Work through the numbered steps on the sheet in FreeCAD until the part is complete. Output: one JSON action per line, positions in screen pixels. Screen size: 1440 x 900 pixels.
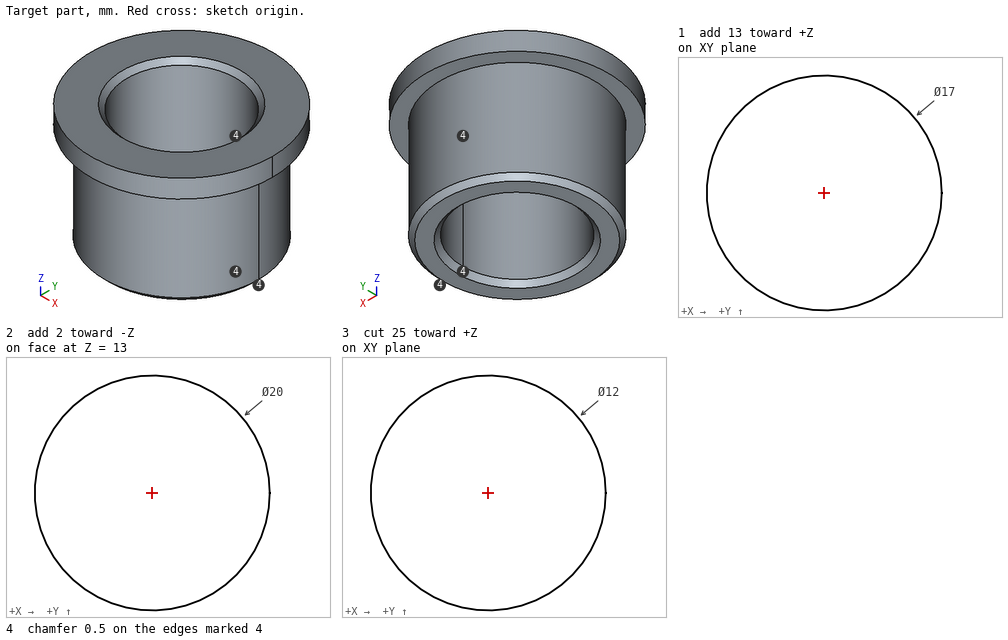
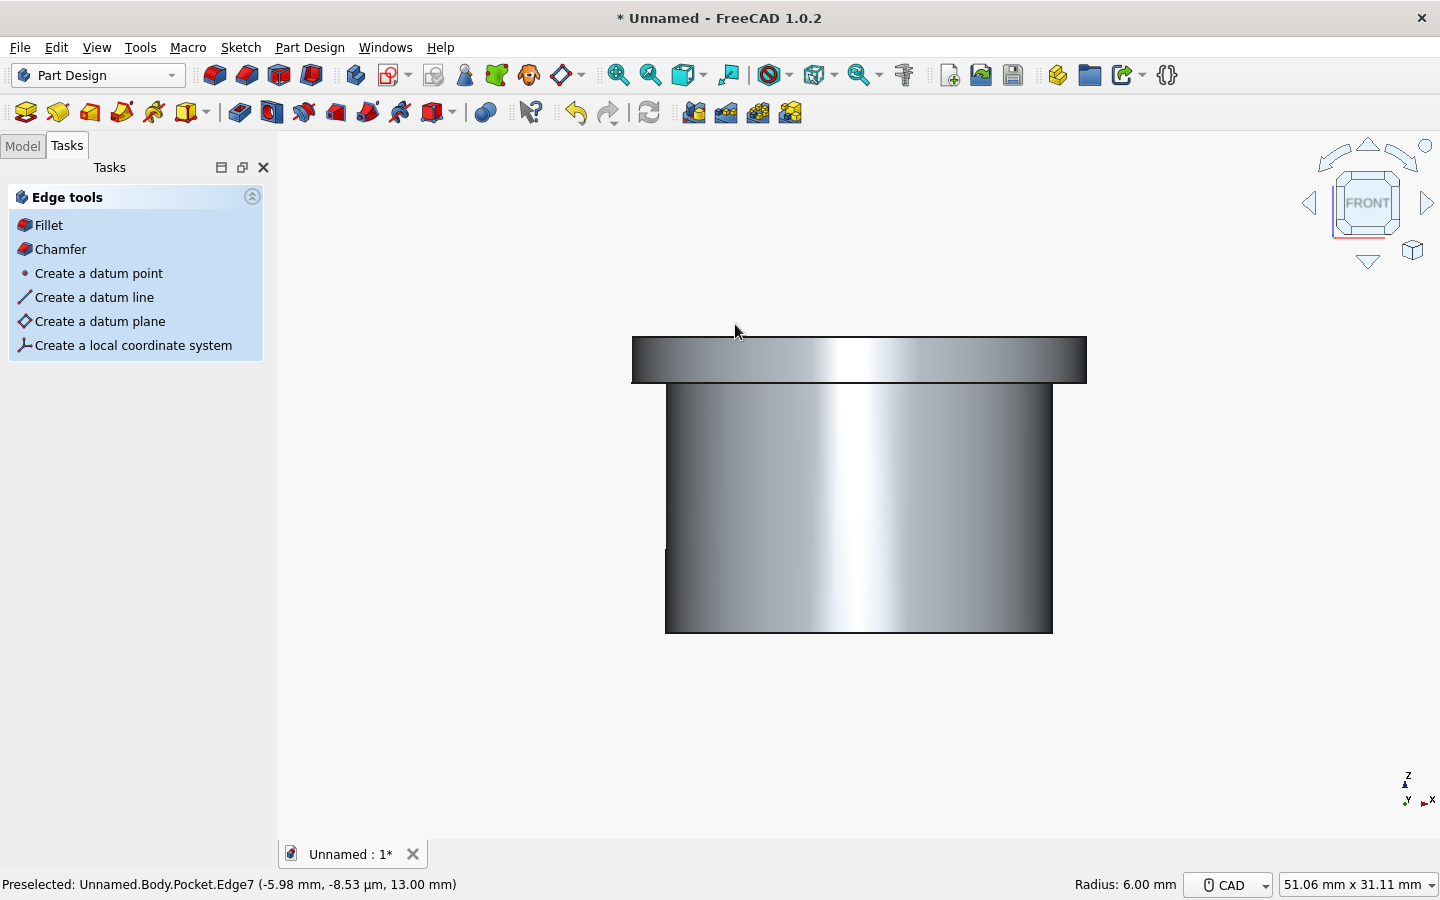
{"action": "key", "text": "v f"}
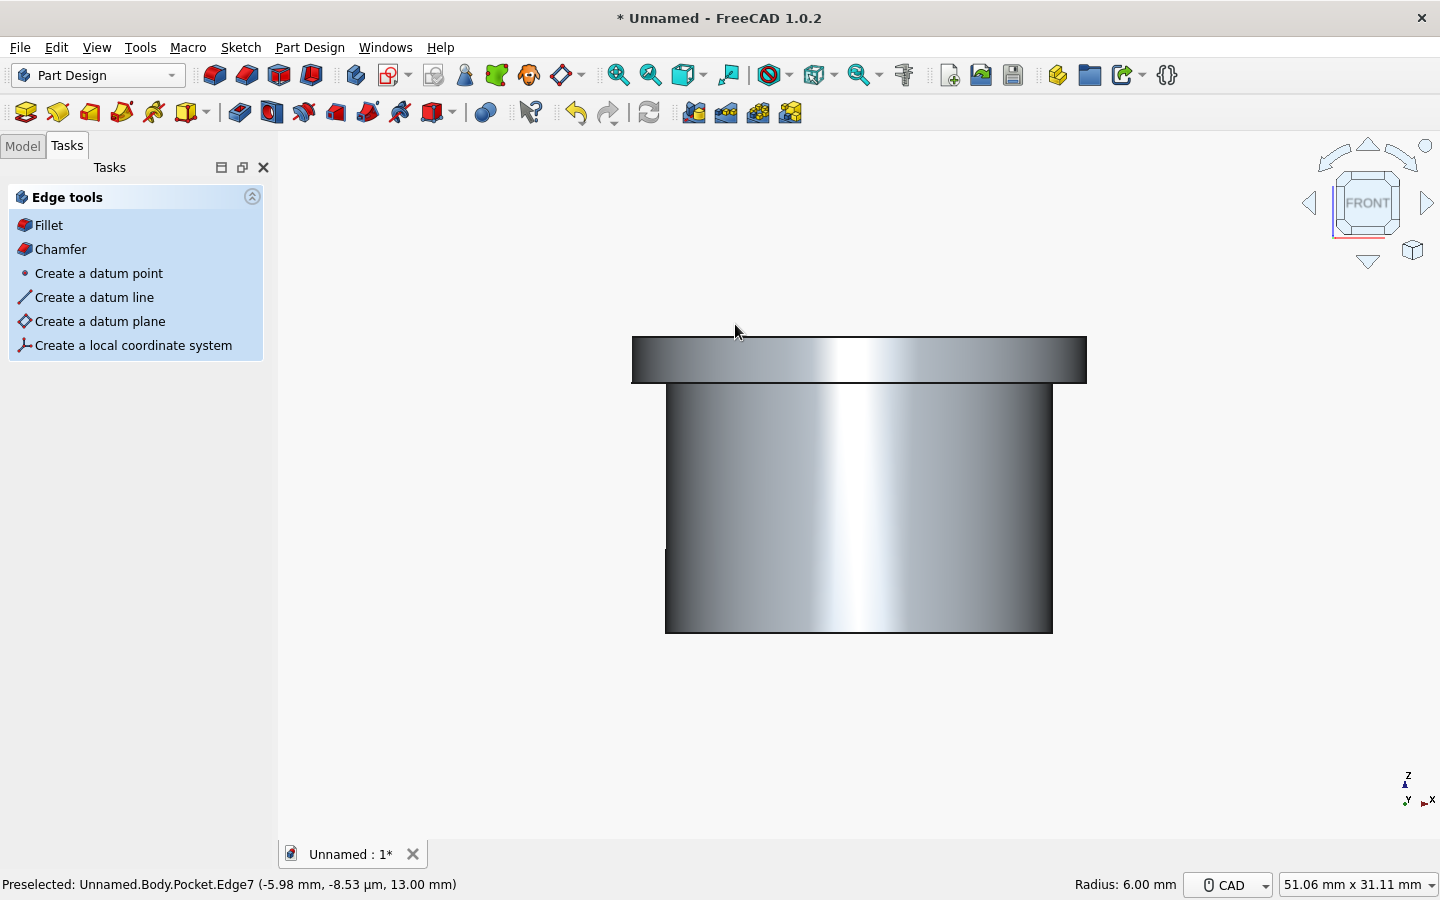
{"action": "key", "text": "3"}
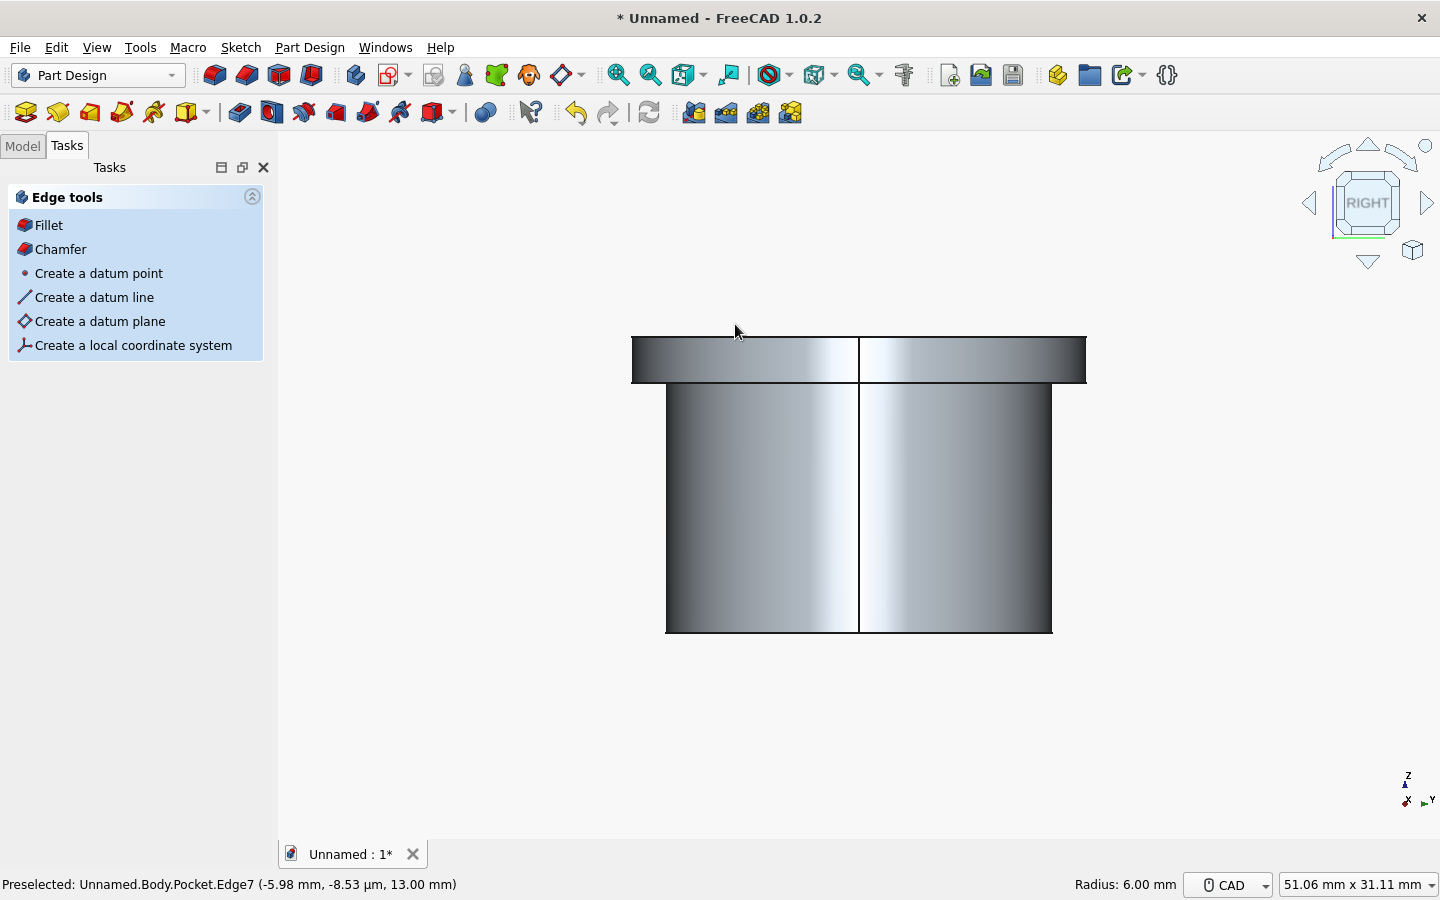
{"action": "left_click", "coordinate": [620, 76]}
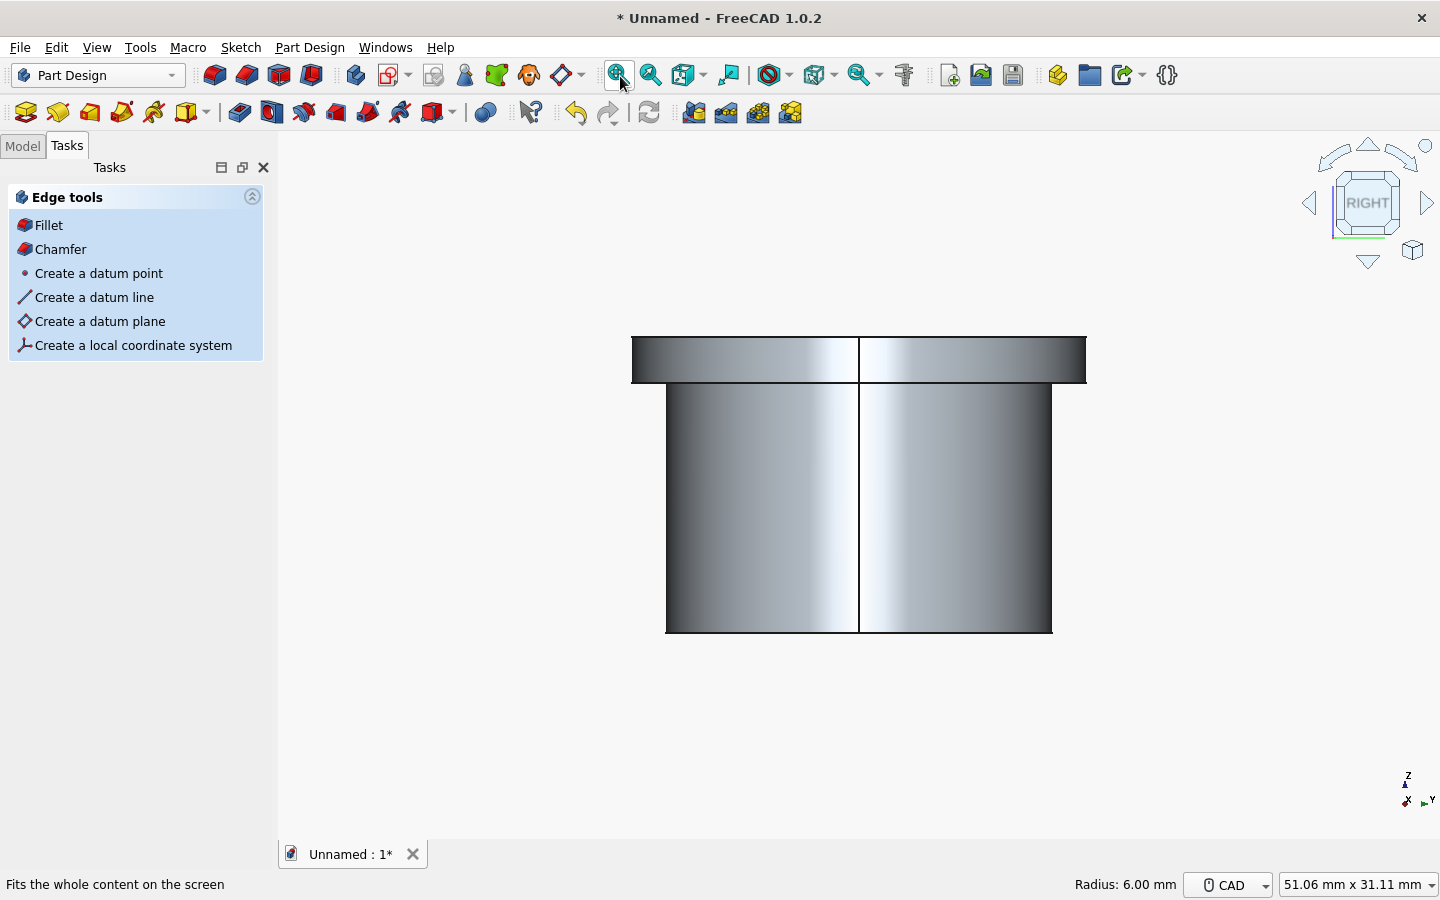
{"action": "key", "text": "5"}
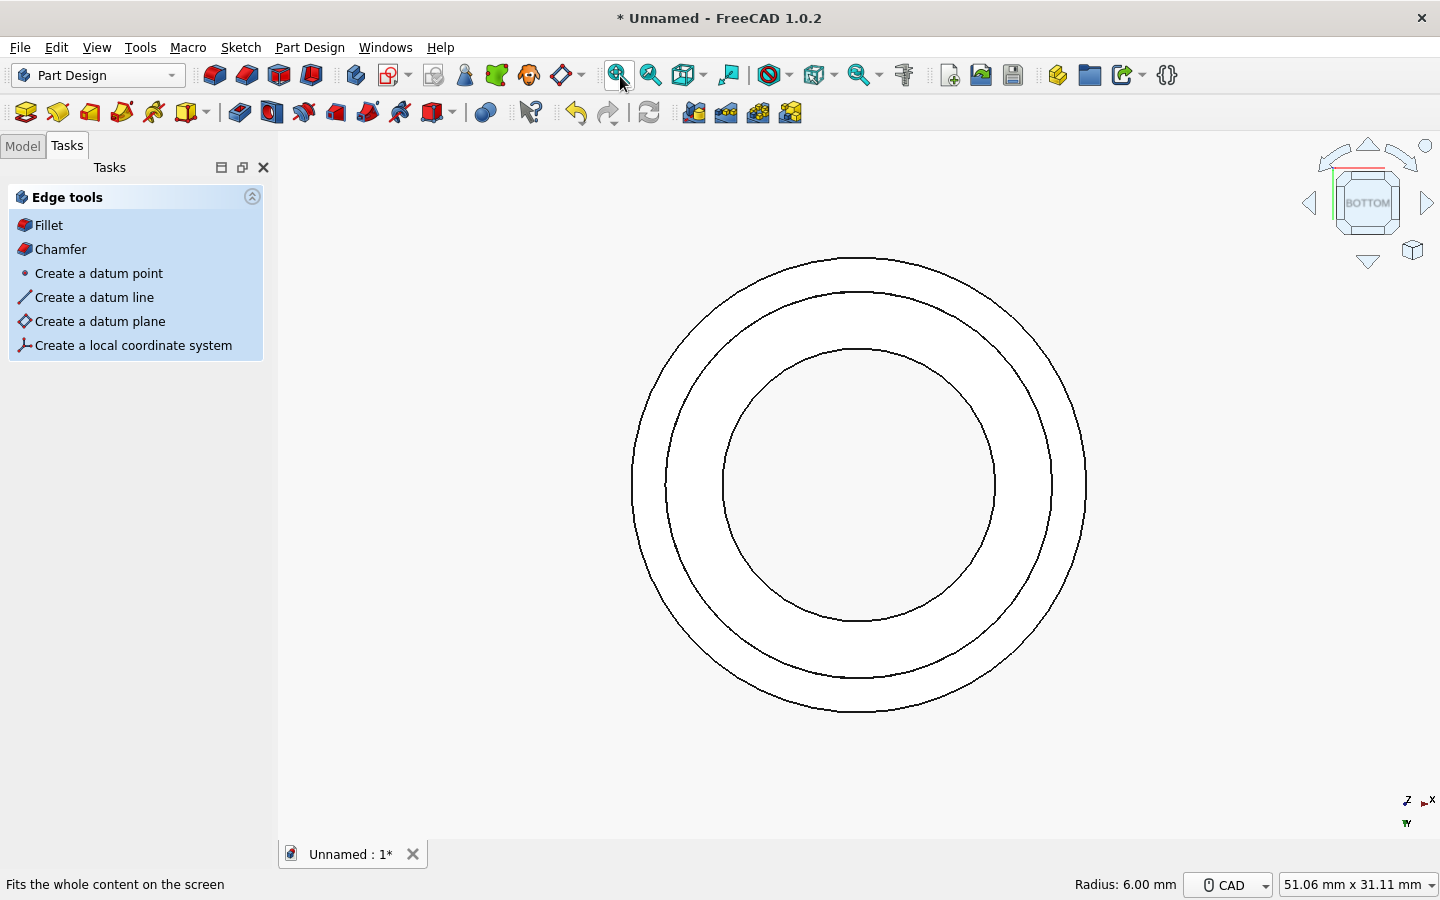
{"action": "left_click", "coordinate": [722, 484], "text": "ctrl"}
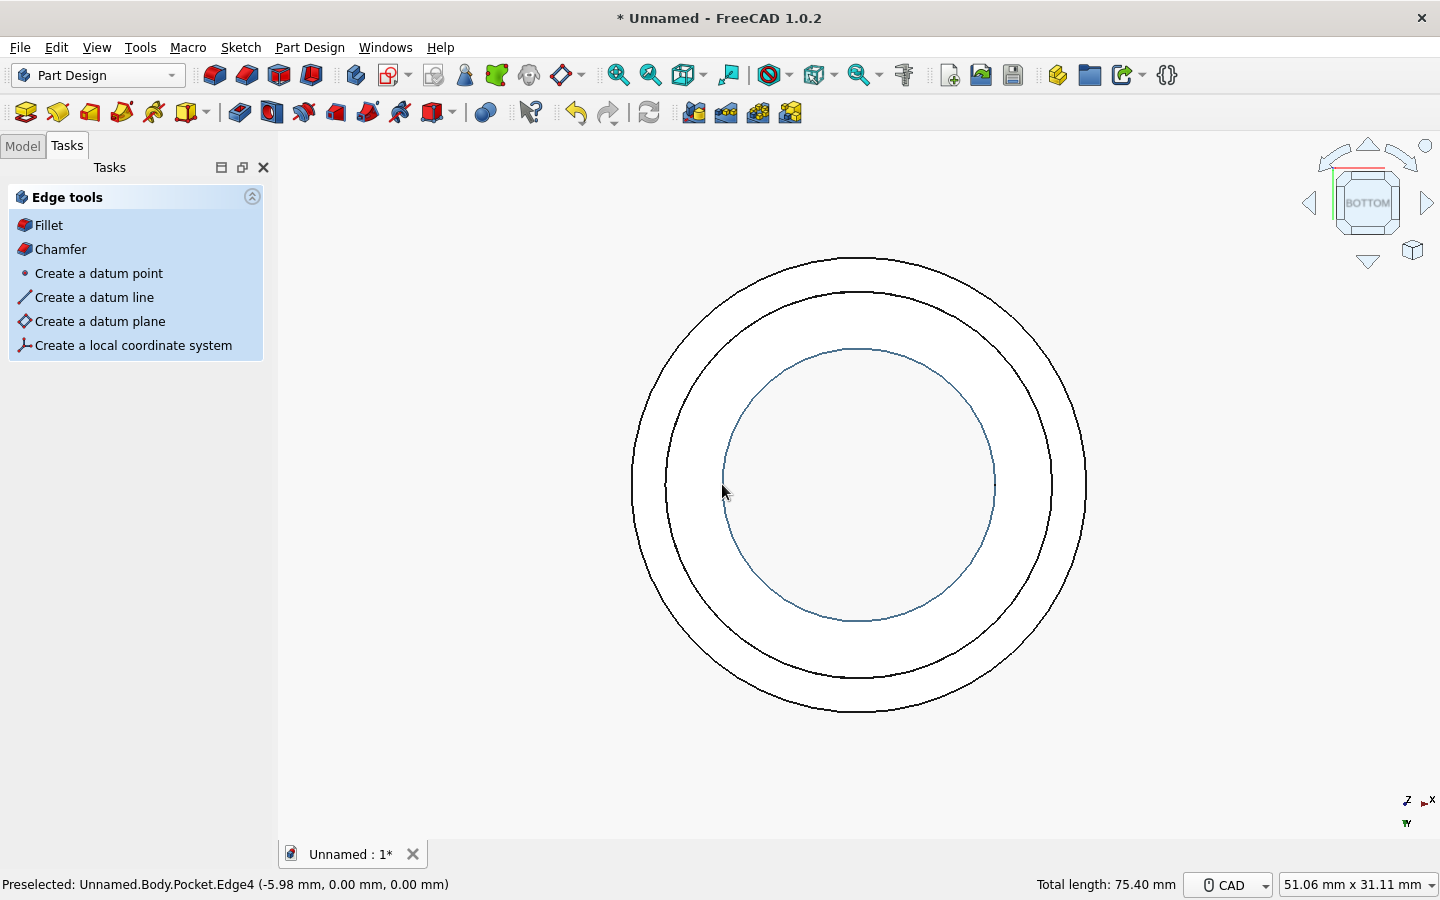
{"action": "left_click", "coordinate": [665, 484], "text": "ctrl"}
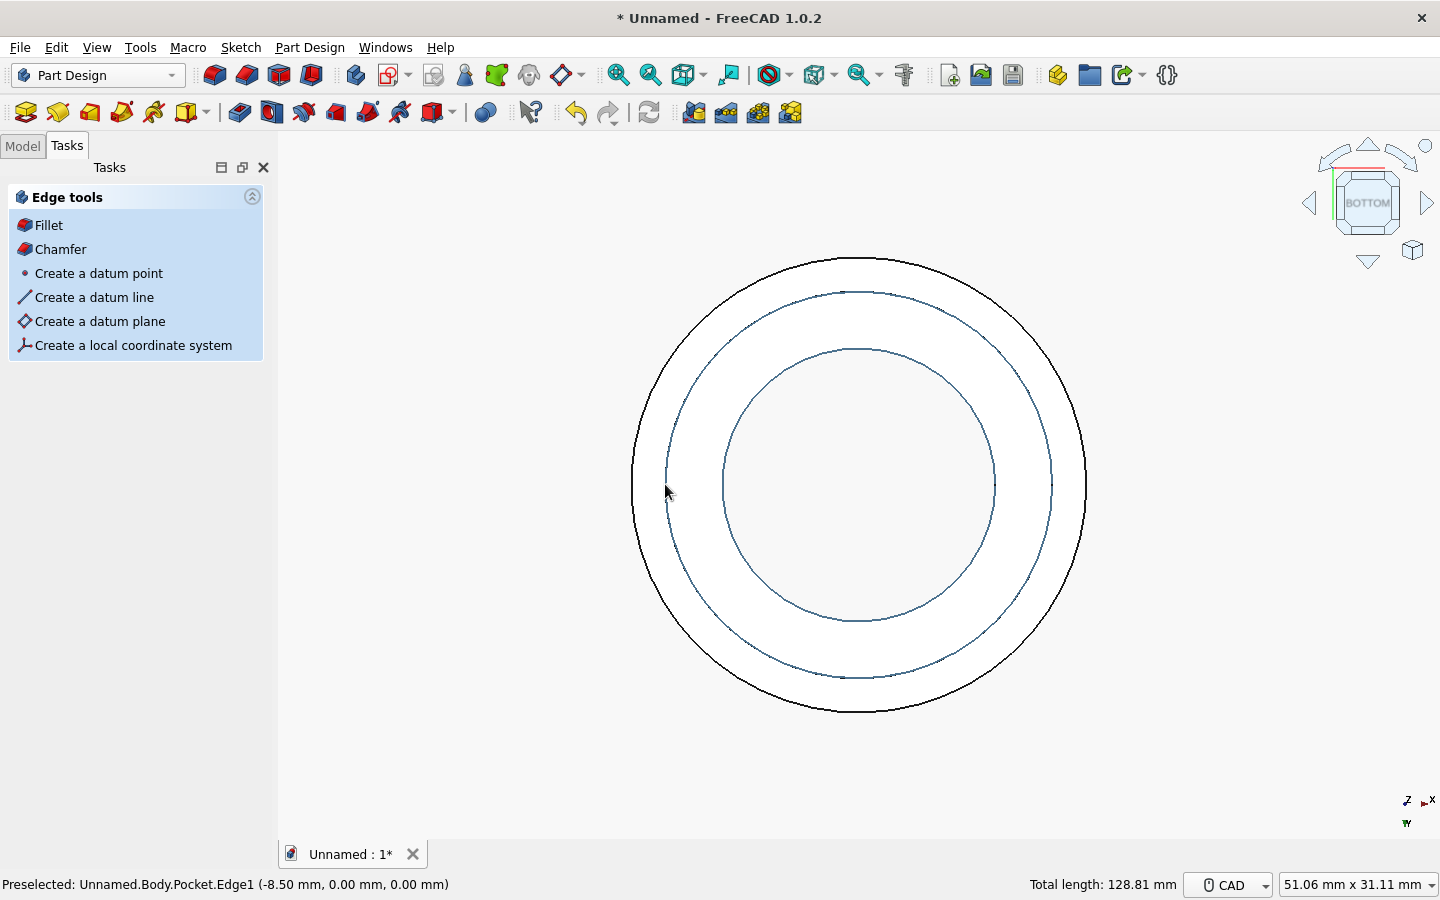
{"action": "left_click", "coordinate": [248, 76]}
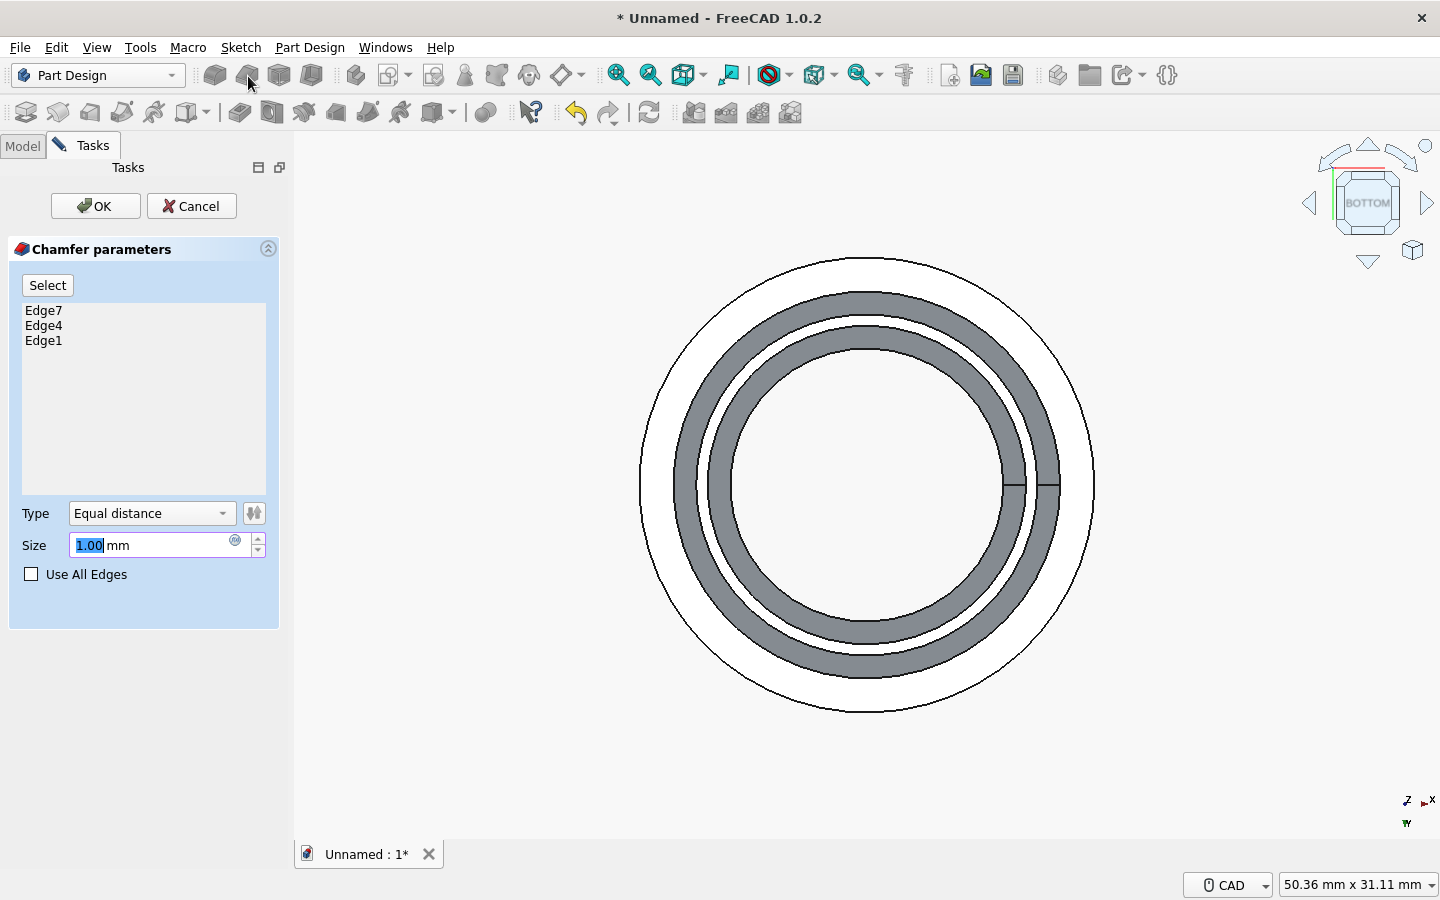
{"action": "type", "text": "0.5"}
{"action": "key", "text": "Tab"}